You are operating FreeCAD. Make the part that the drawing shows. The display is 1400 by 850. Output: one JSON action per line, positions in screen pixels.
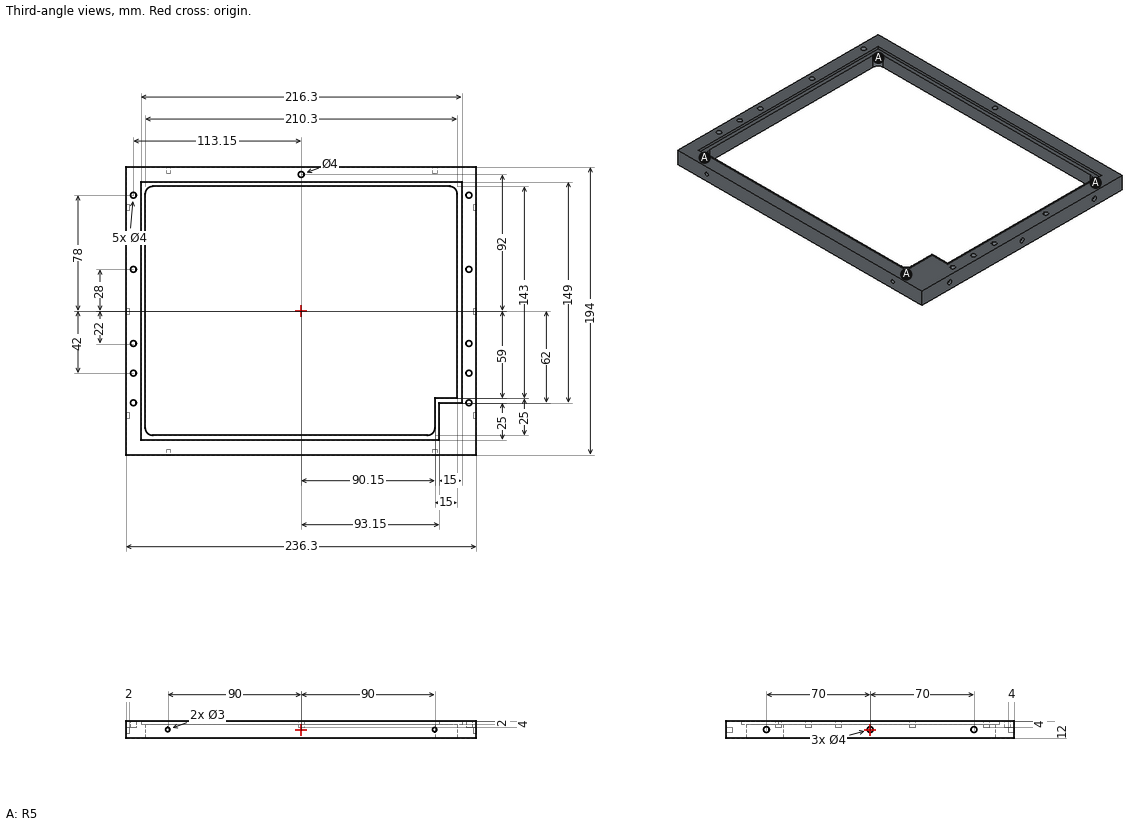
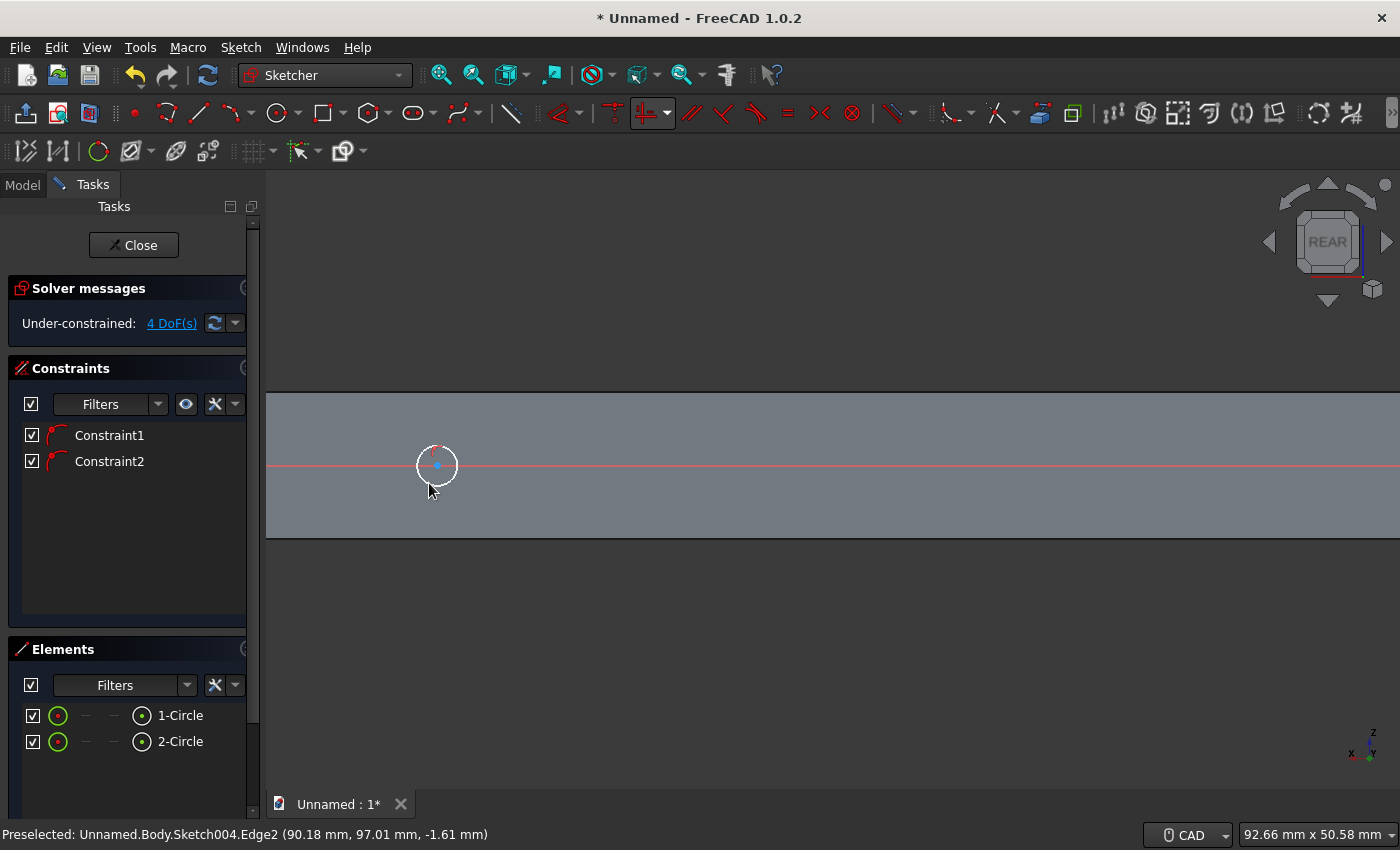
{"action": "scroll", "coordinate": [431, 485], "scroll_direction": "down", "scroll_amount": 6}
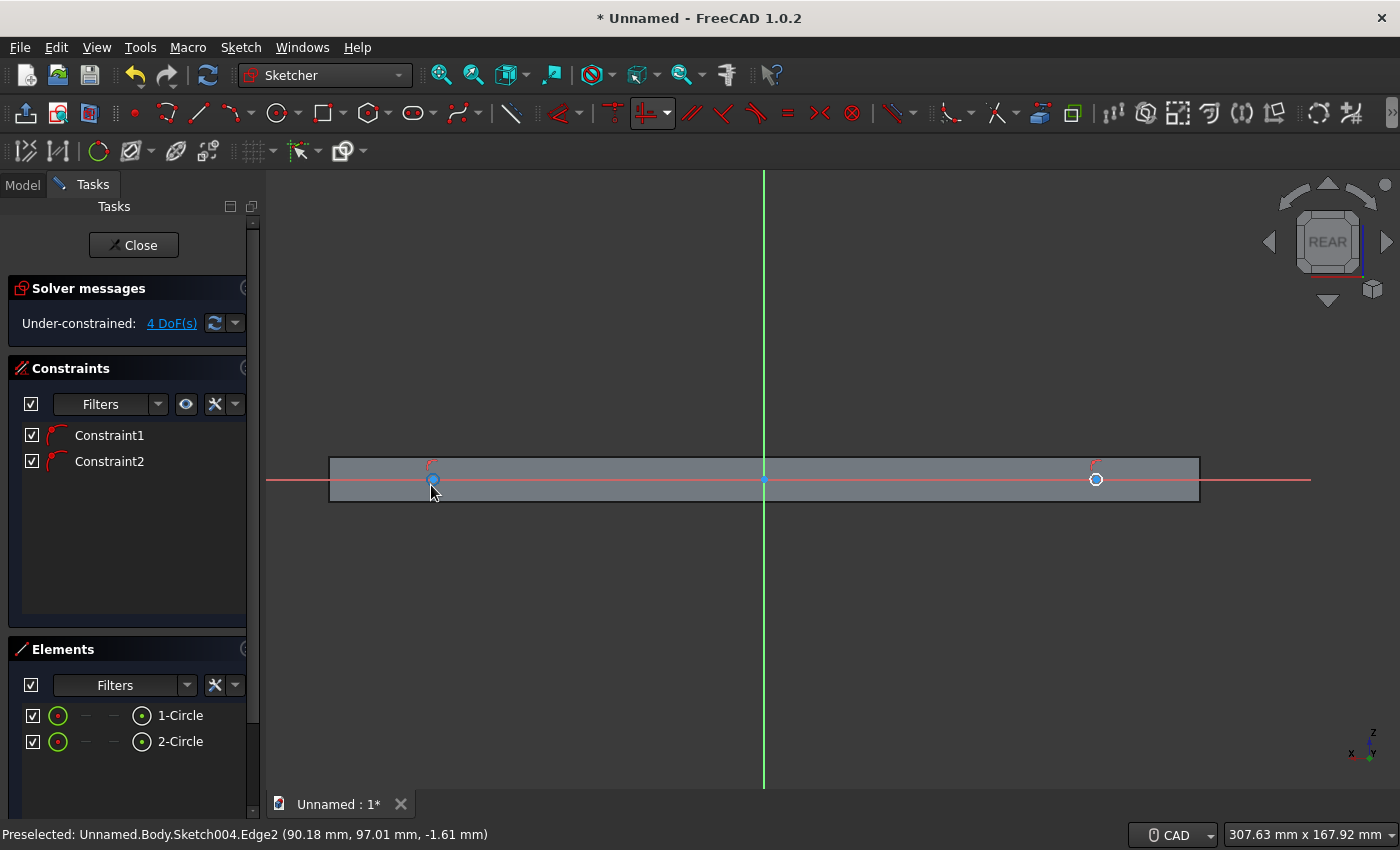
{"action": "scroll", "coordinate": [1100, 475], "scroll_direction": "up", "scroll_amount": 7}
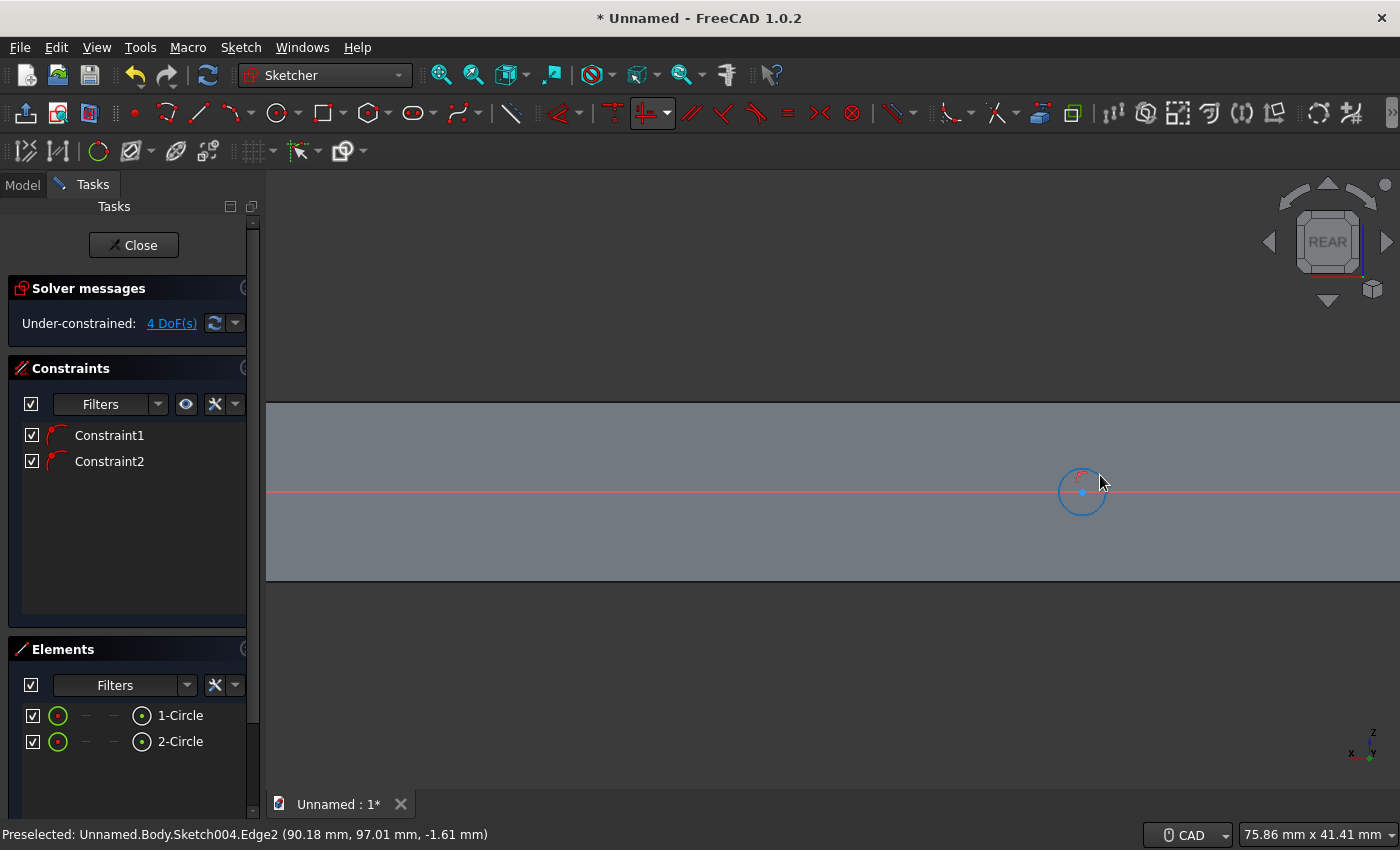
{"action": "left_click", "coordinate": [1099, 475]}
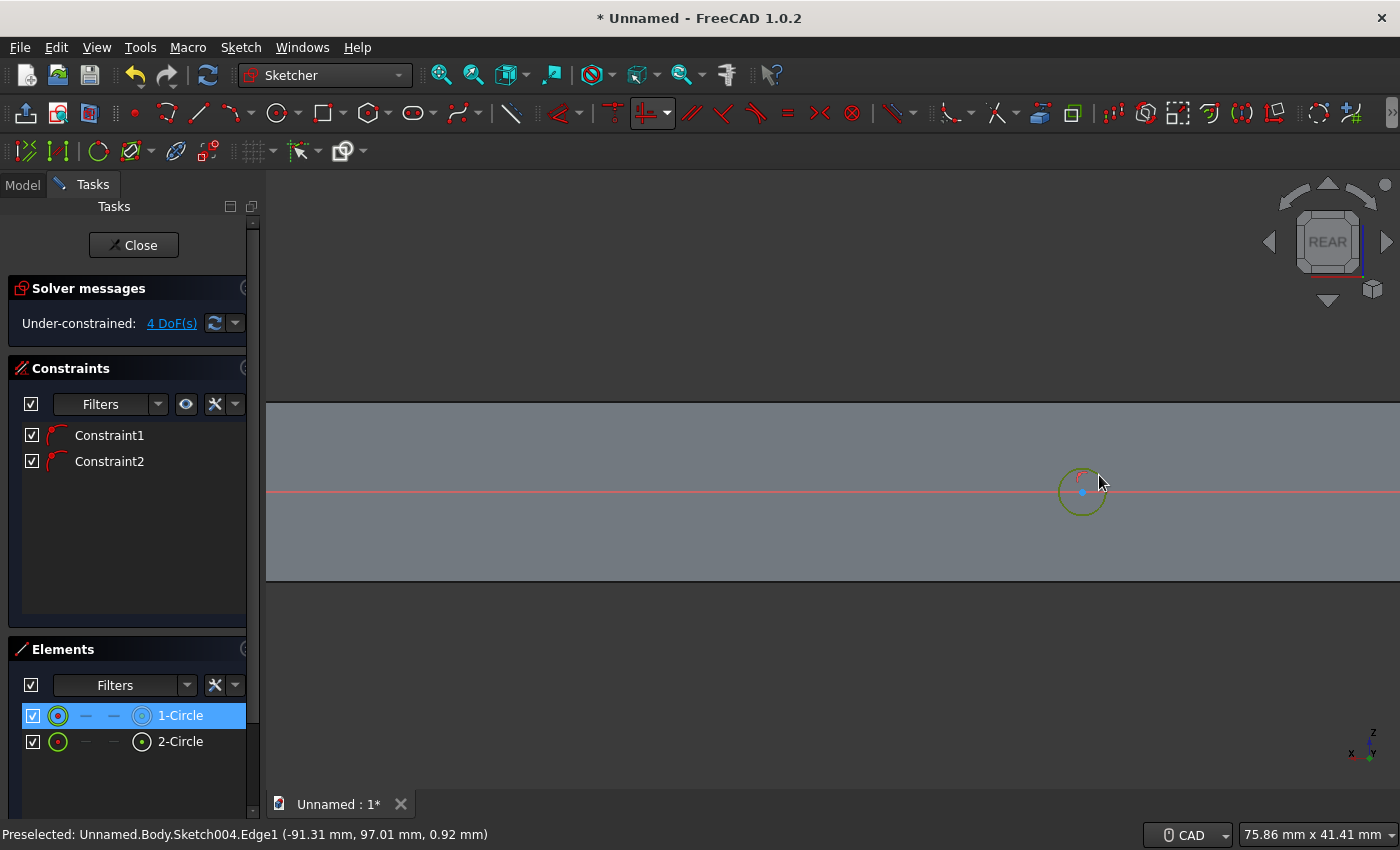
{"action": "scroll", "coordinate": [1101, 475], "scroll_direction": "down", "scroll_amount": 7}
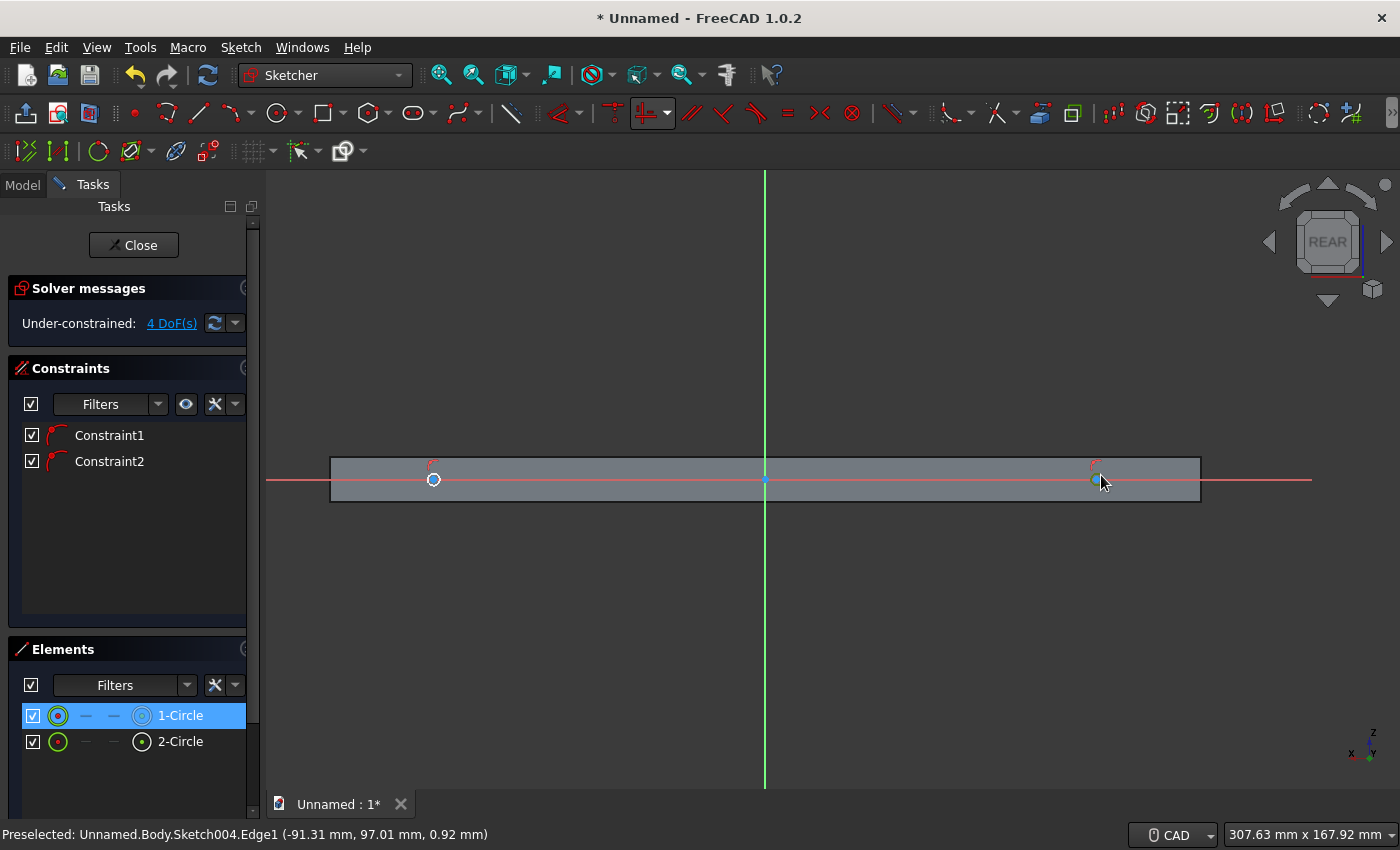
{"action": "scroll", "coordinate": [438, 475], "scroll_direction": "up", "scroll_amount": 6}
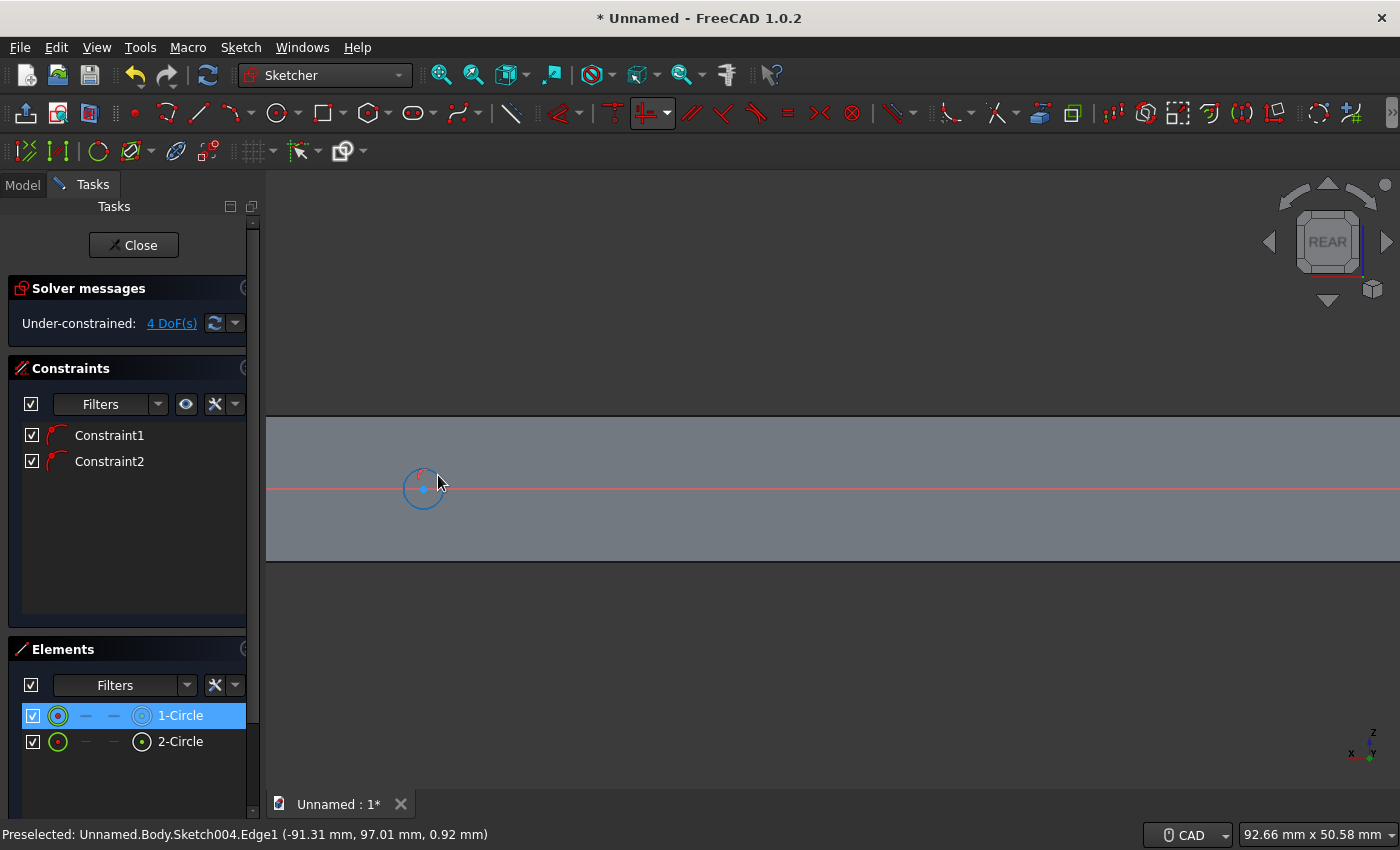
{"action": "left_click", "coordinate": [438, 475]}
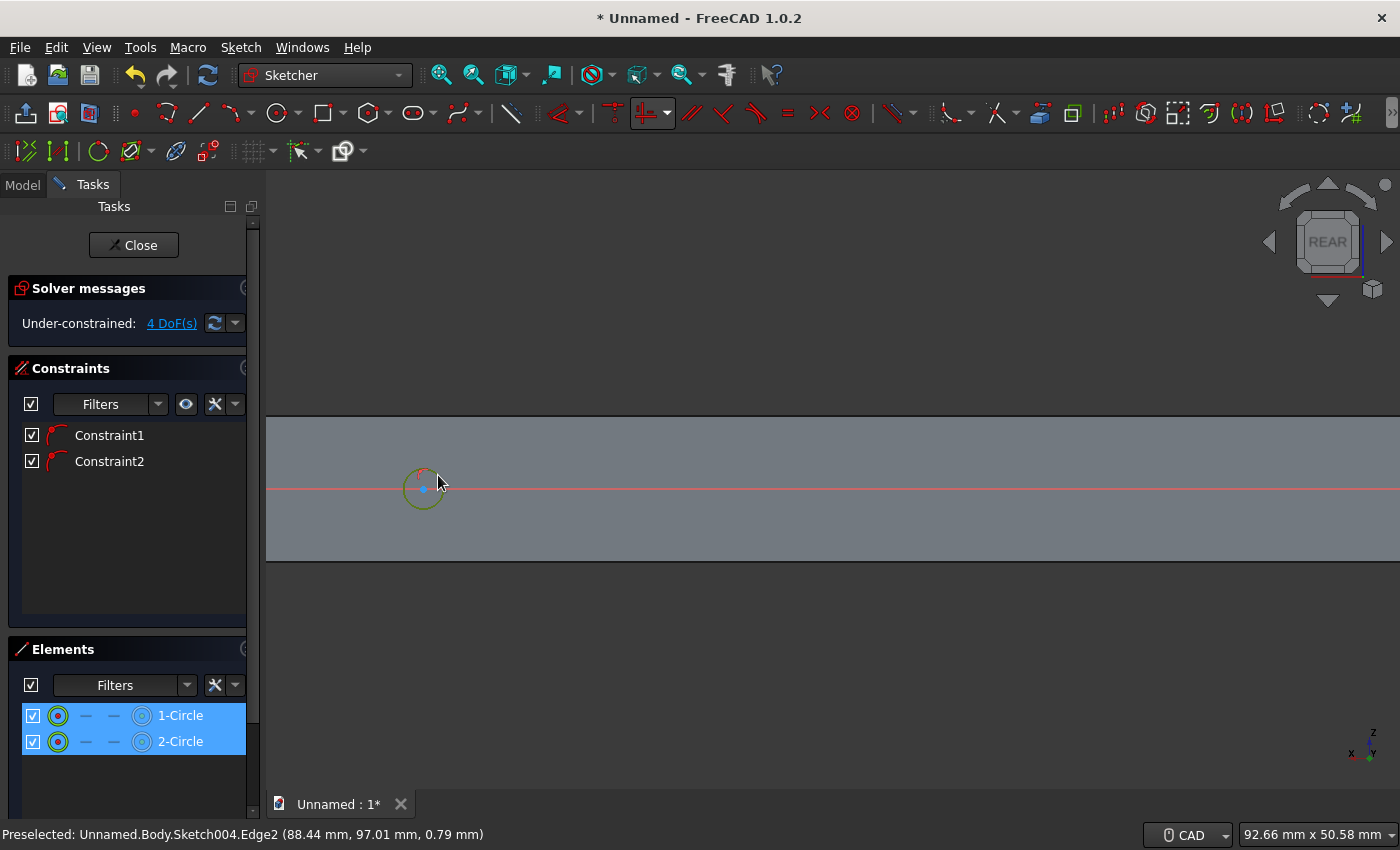
{"action": "left_click", "coordinate": [788, 114]}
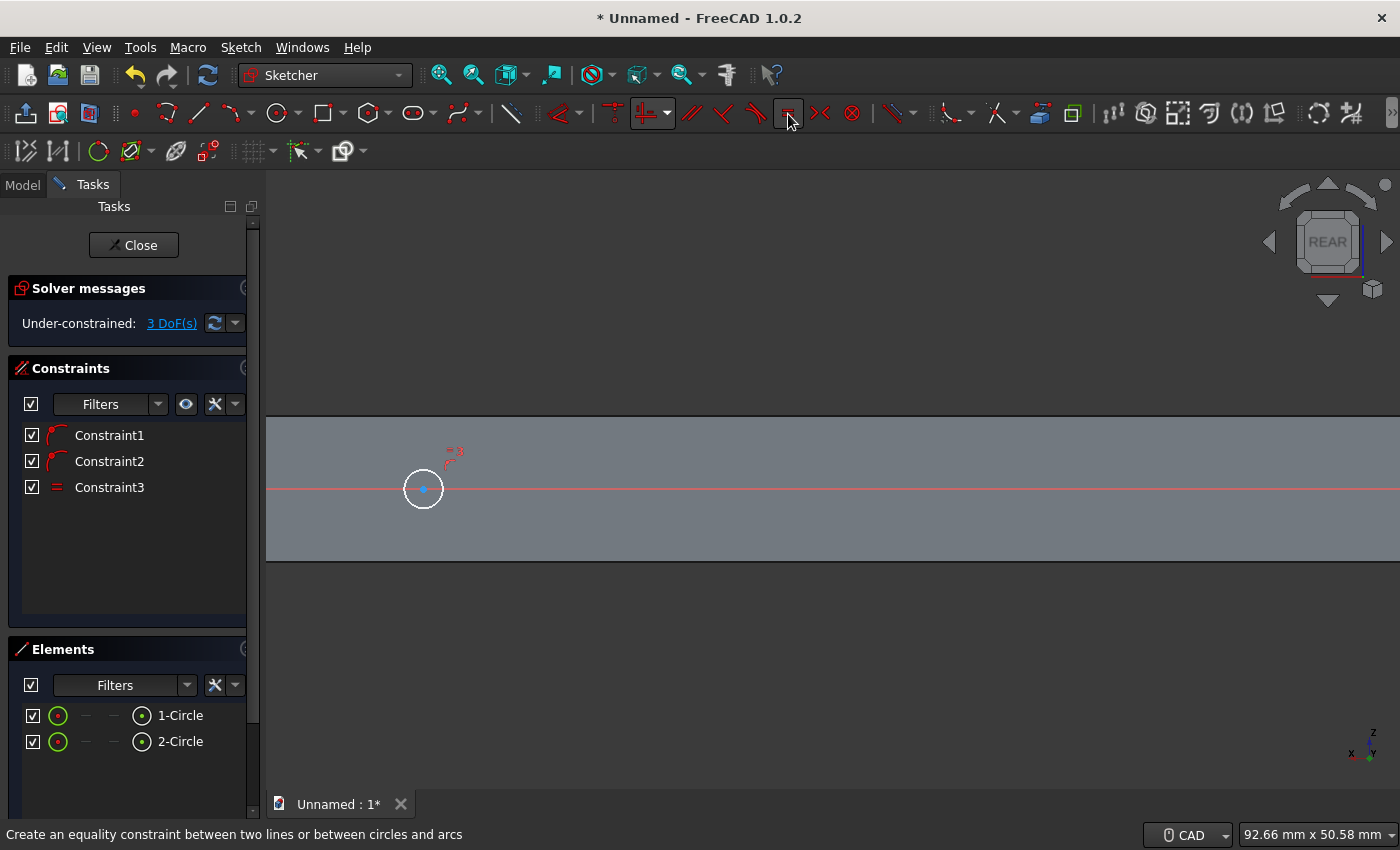
{"action": "left_click", "coordinate": [558, 114]}